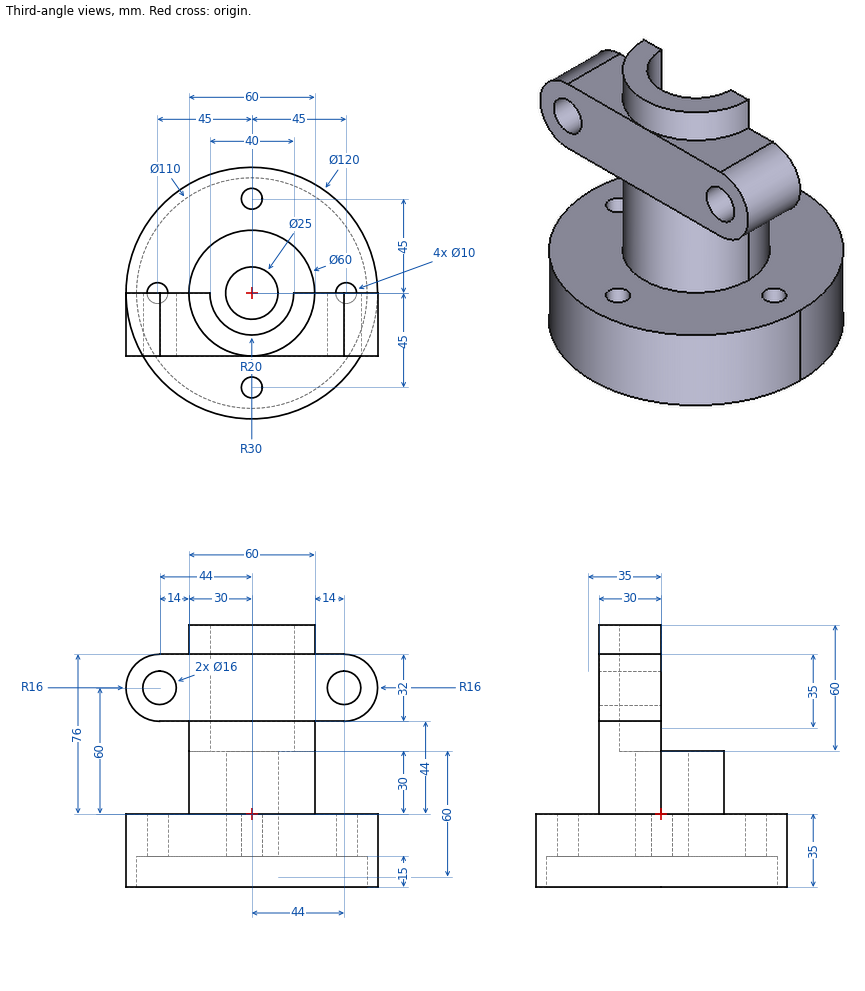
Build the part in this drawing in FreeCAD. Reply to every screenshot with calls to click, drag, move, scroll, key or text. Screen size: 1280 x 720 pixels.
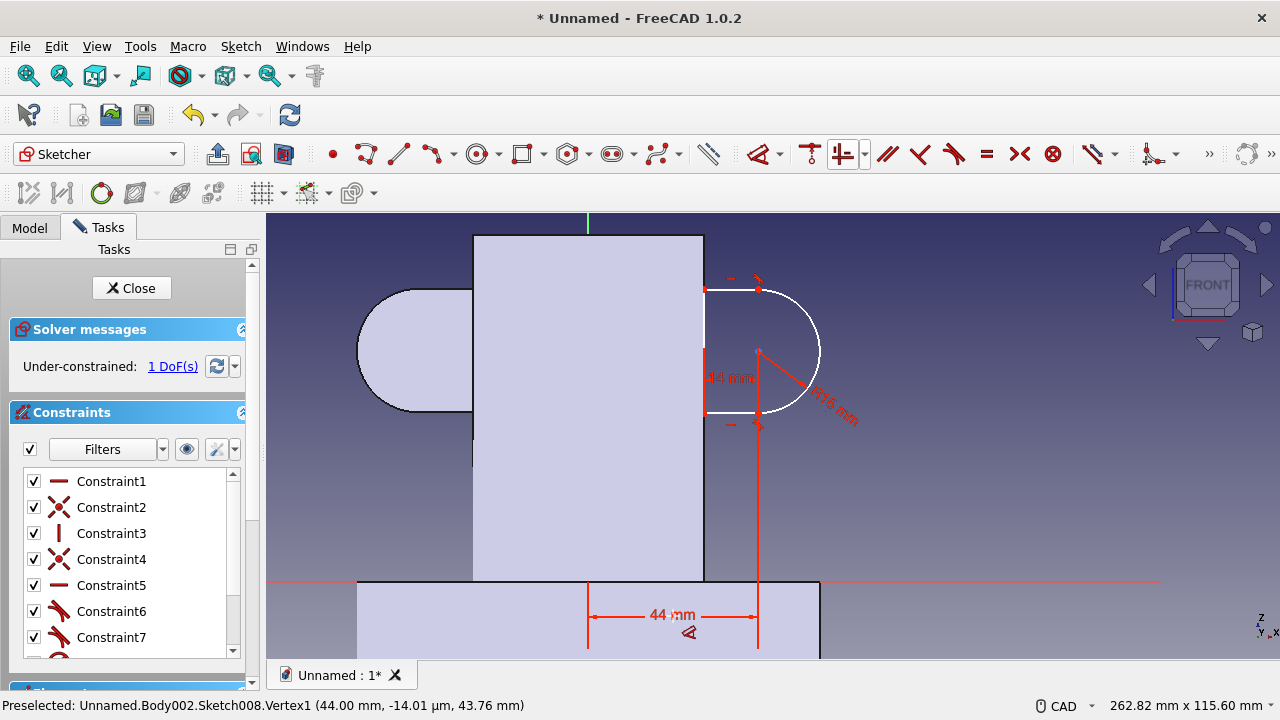
click(758, 413)
click(554, 498)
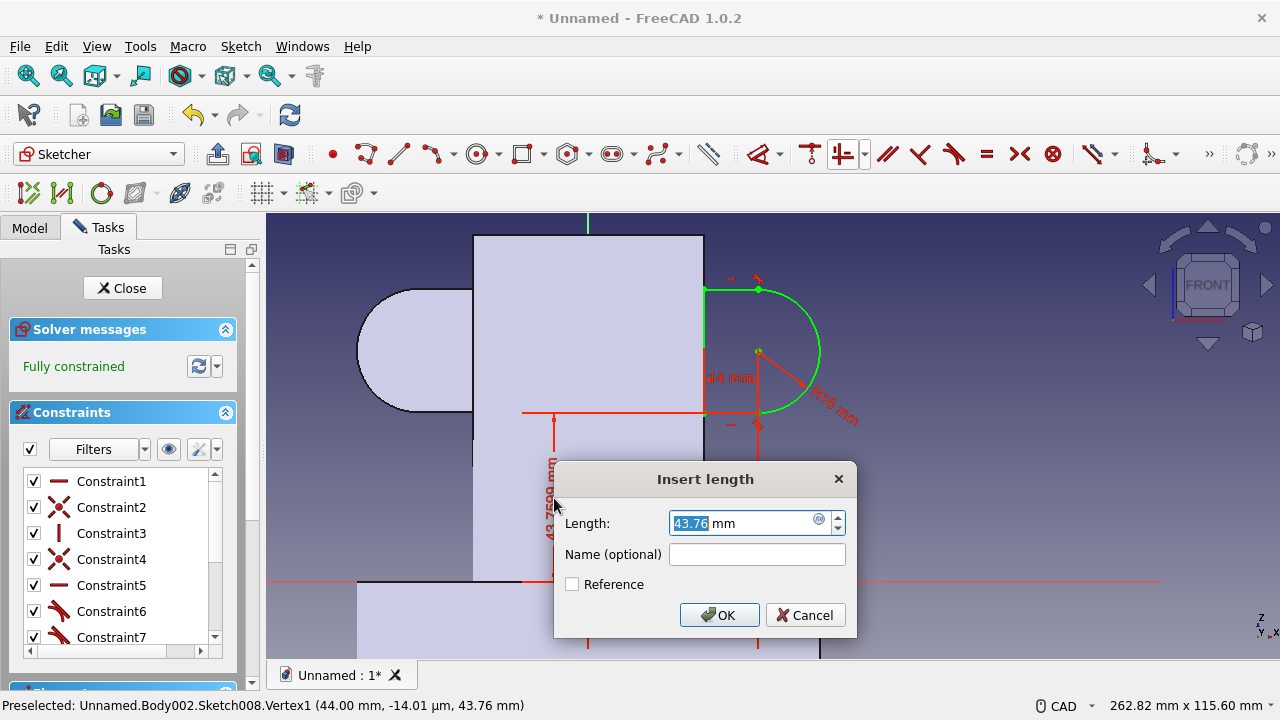
text(44)
key(Return)
key(Escape)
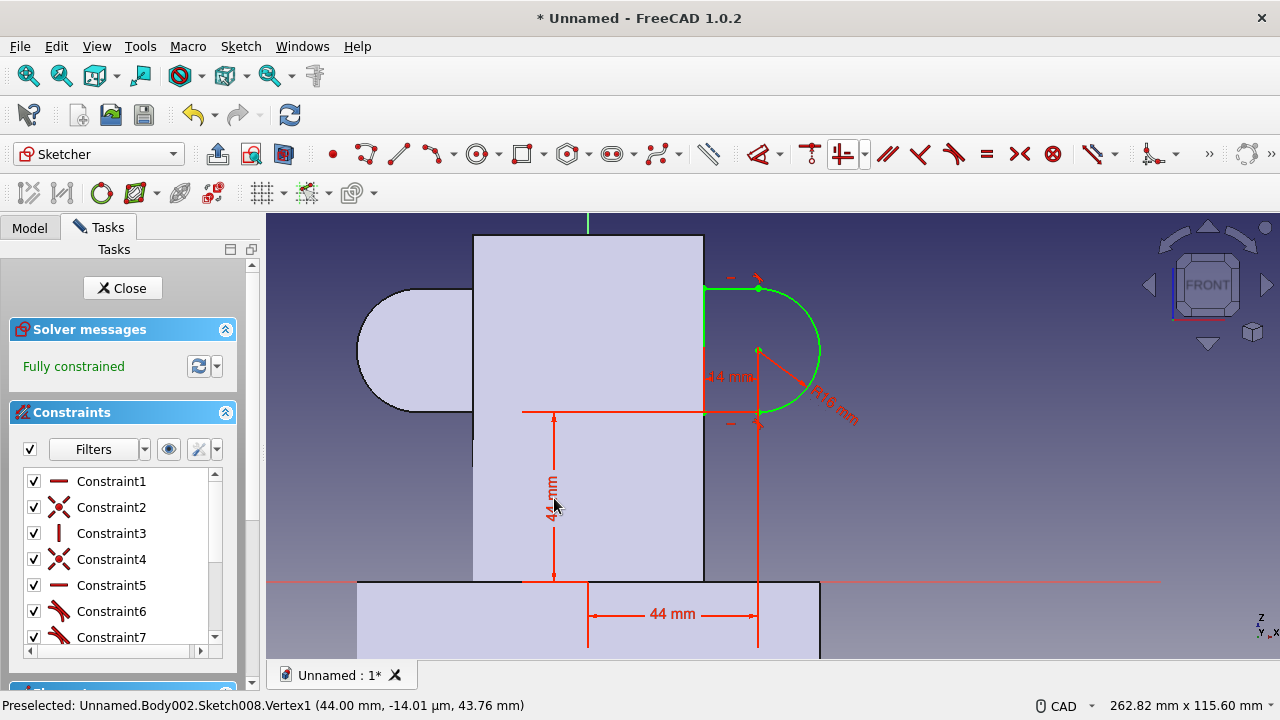
click(123, 288)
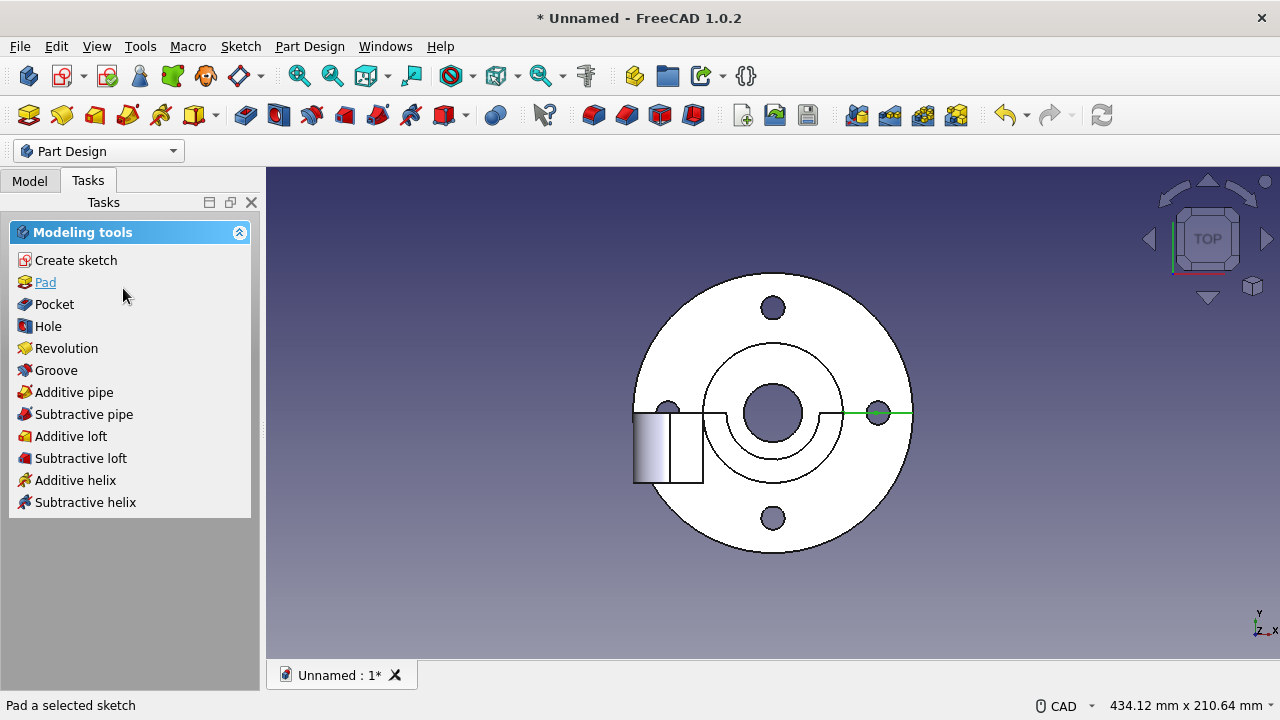
click(29, 116)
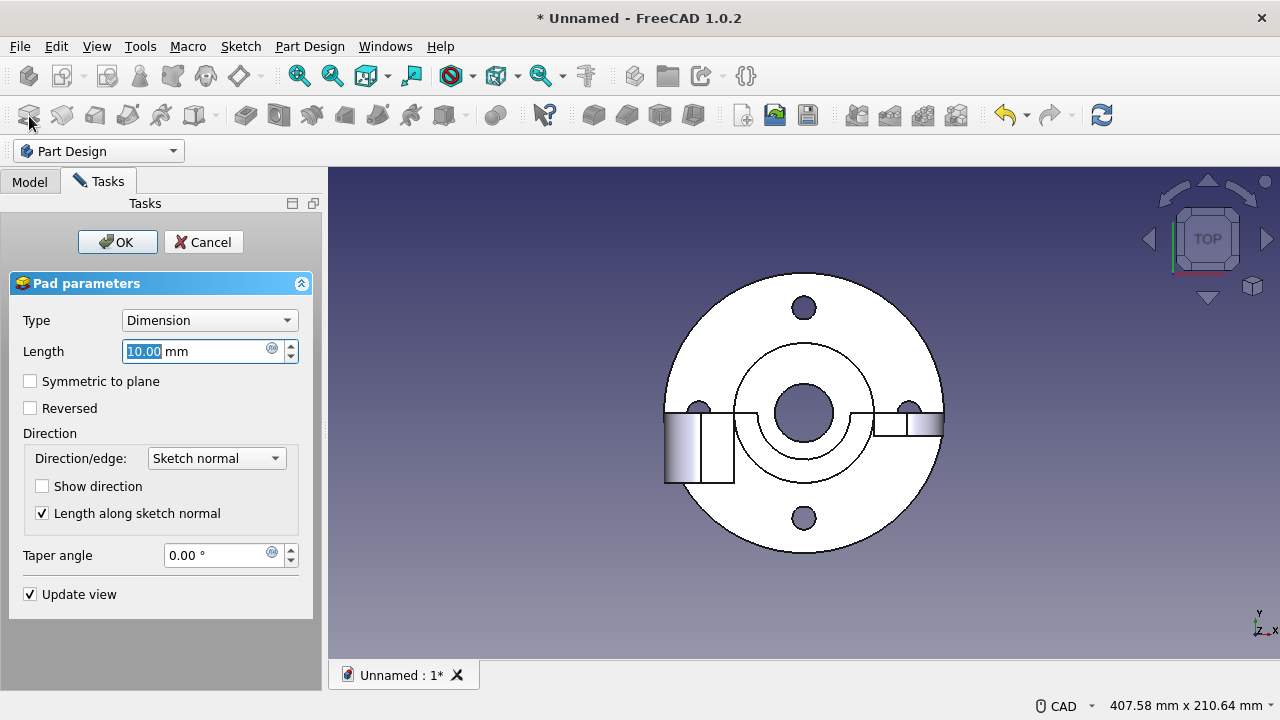
text(30)
key(Tab)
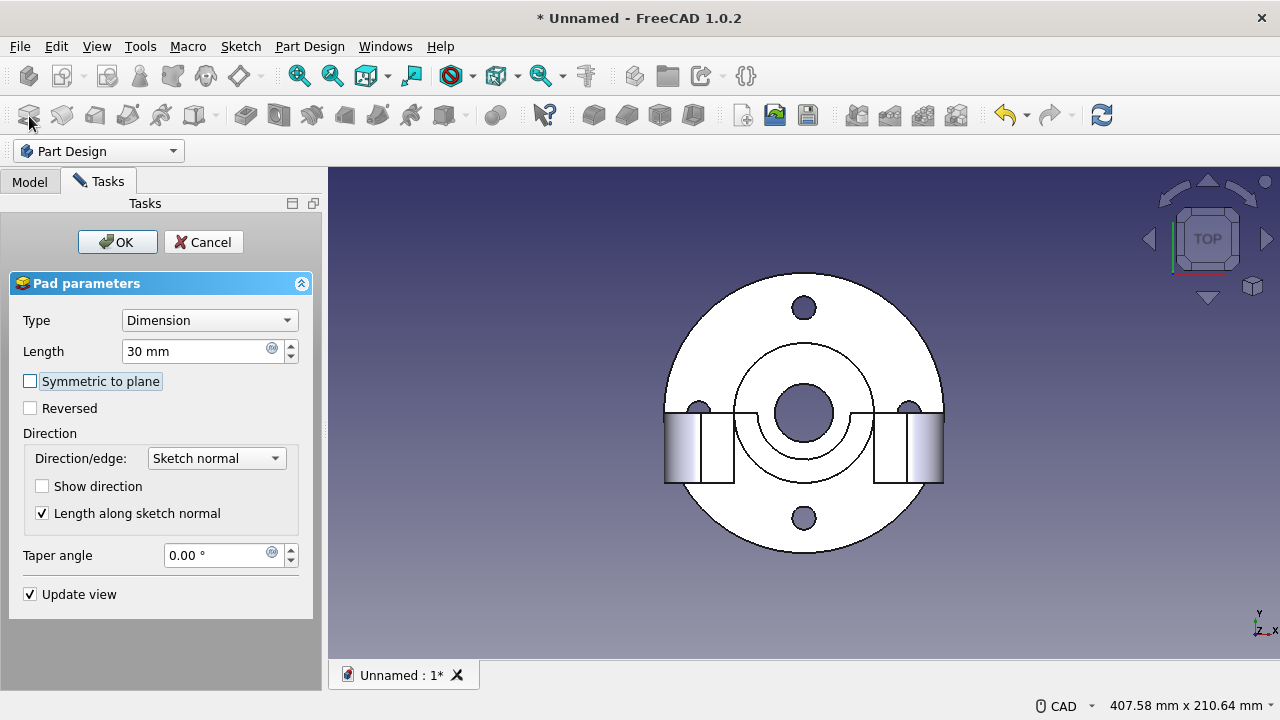
click(118, 242)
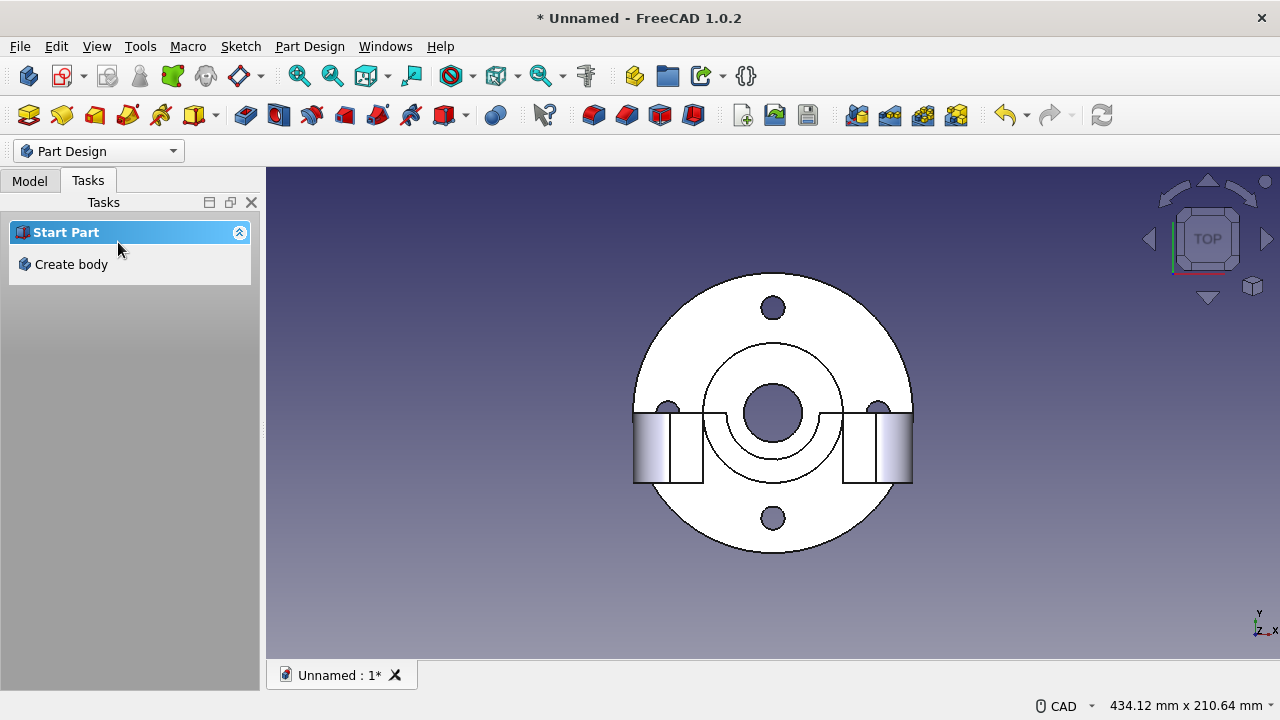
click(300, 76)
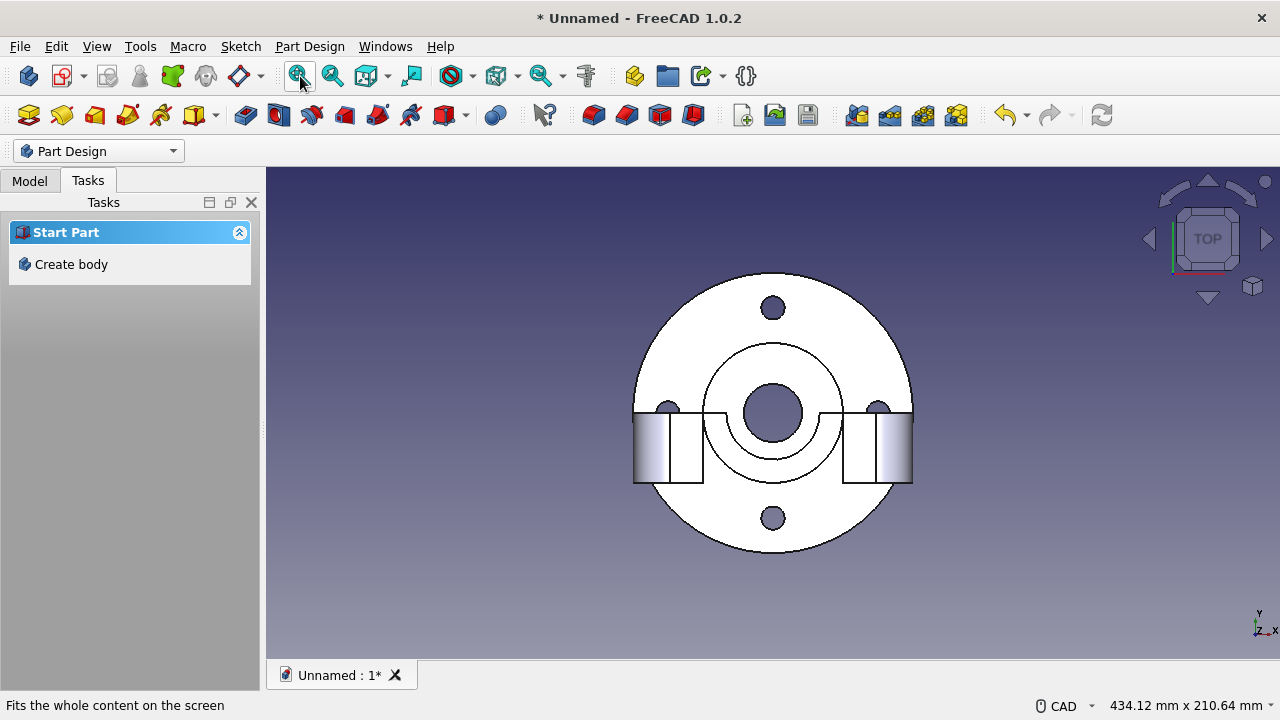
click(30, 180)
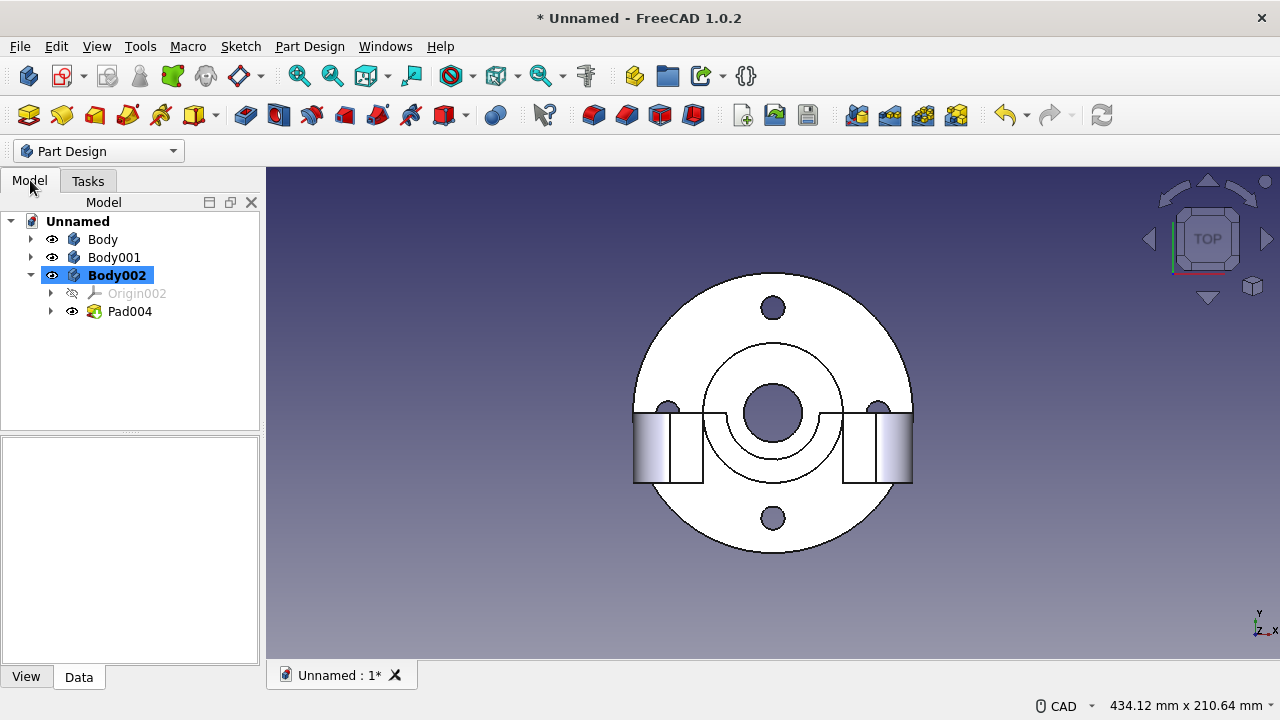
double_click(97, 239)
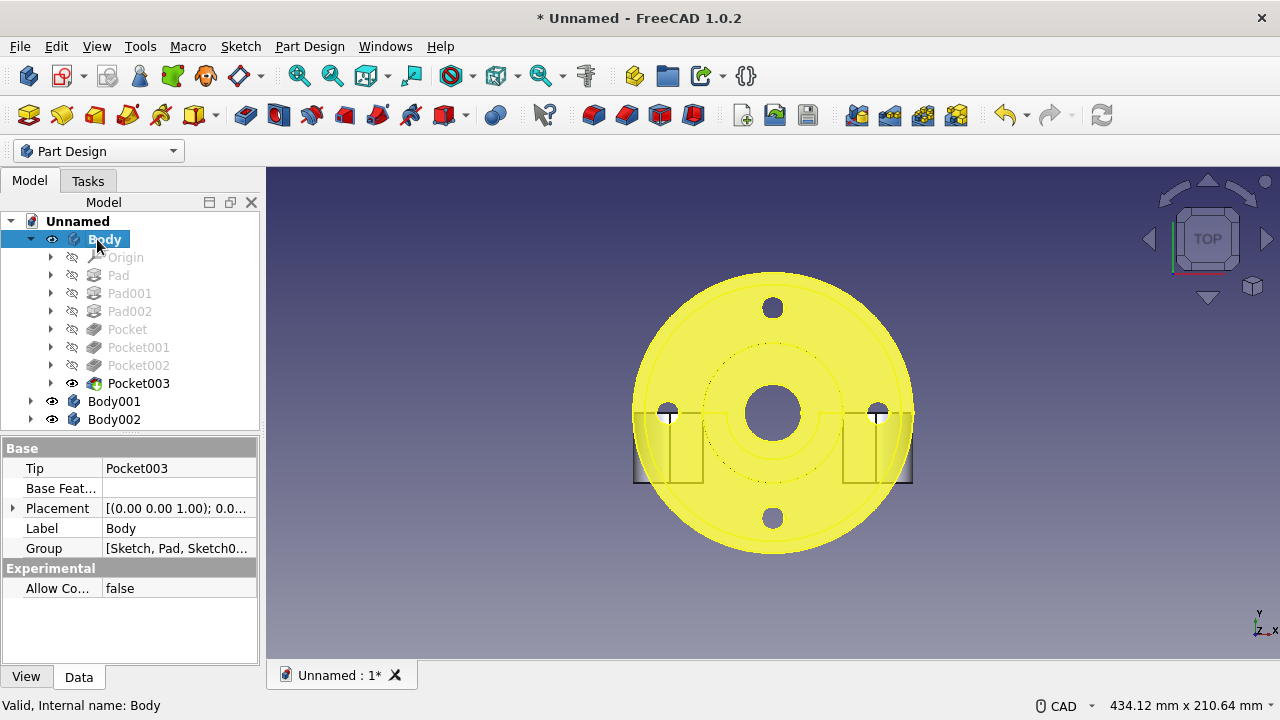
click(97, 239)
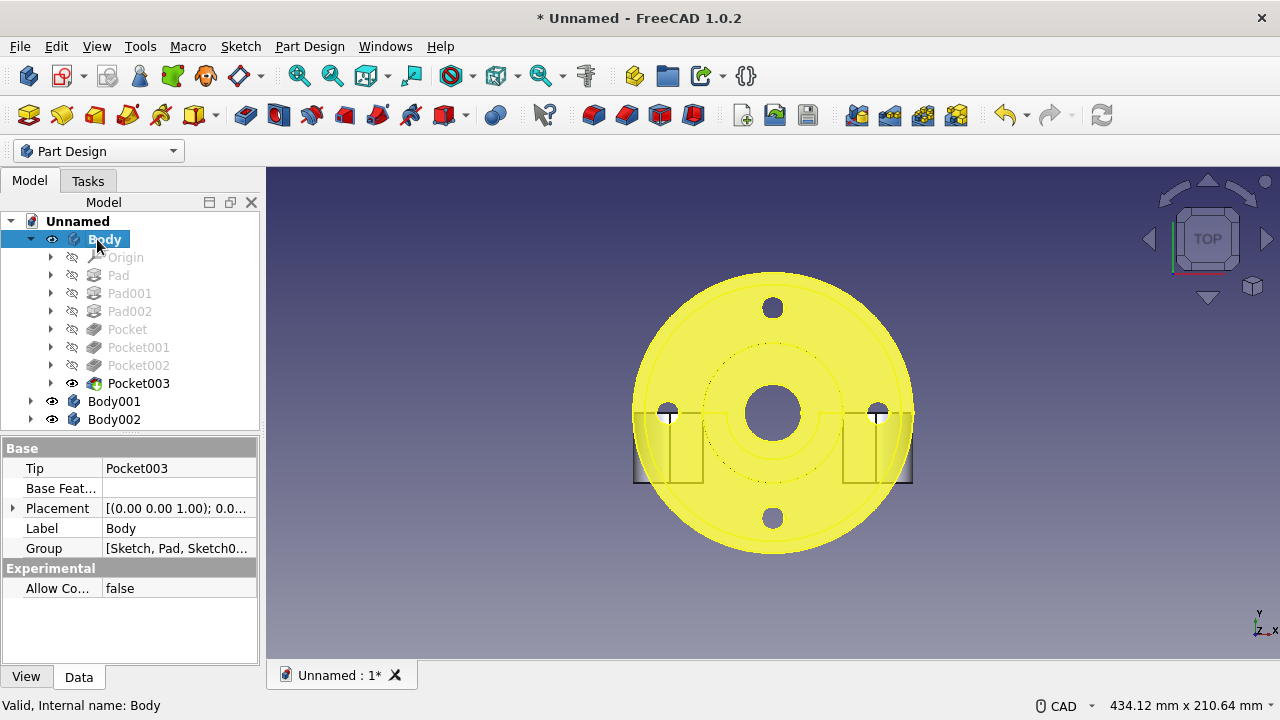
click(148, 588)